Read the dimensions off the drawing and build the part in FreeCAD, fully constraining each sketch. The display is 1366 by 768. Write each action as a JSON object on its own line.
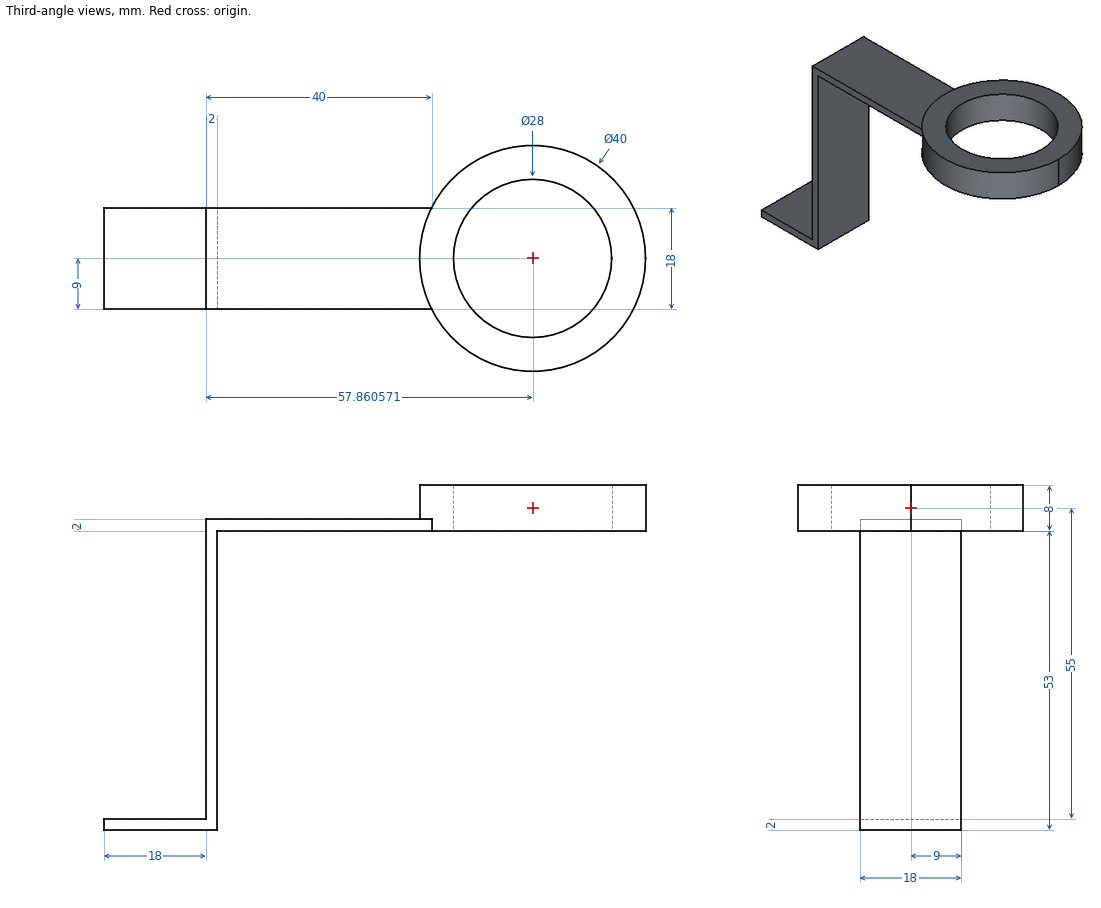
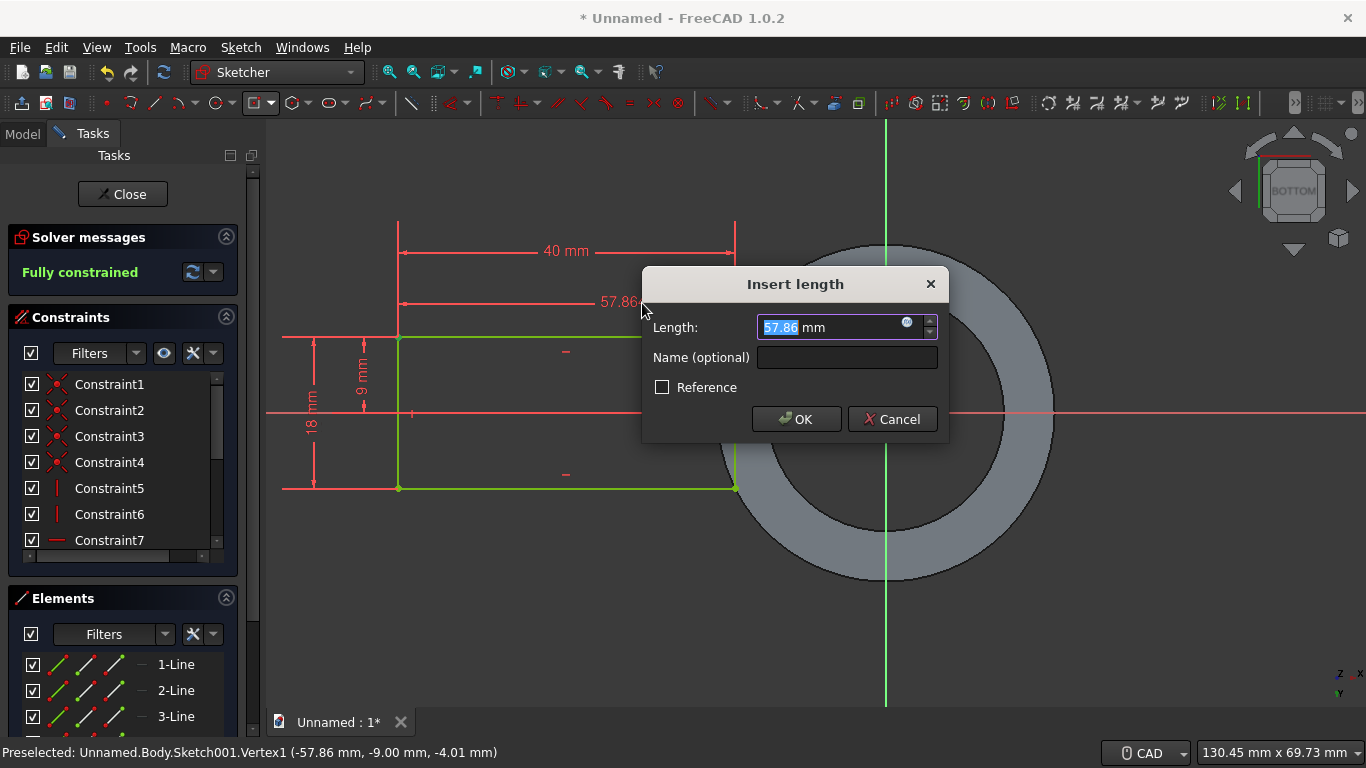
{"action": "type", "text": "57.860571"}
{"action": "key", "text": "Return"}
{"action": "key", "text": "Escape"}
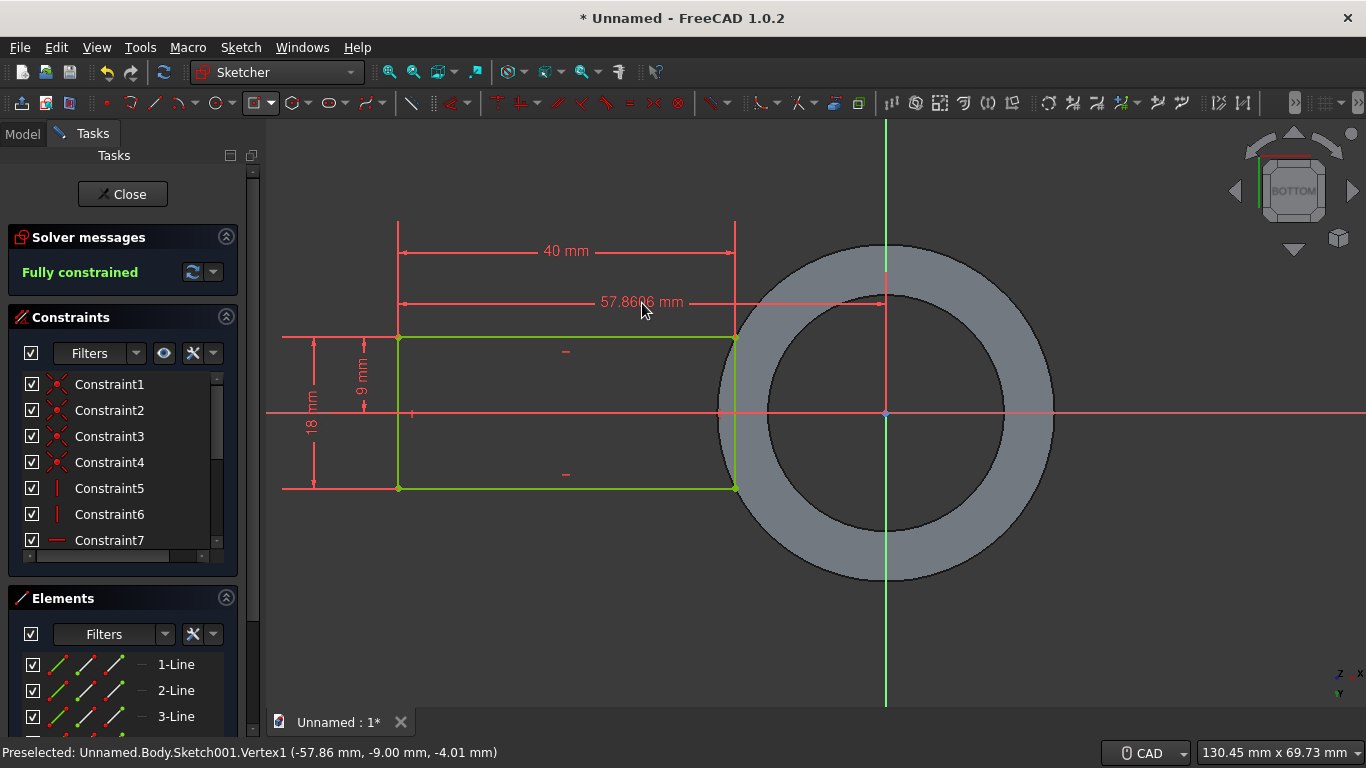
{"action": "left_click", "coordinate": [123, 194]}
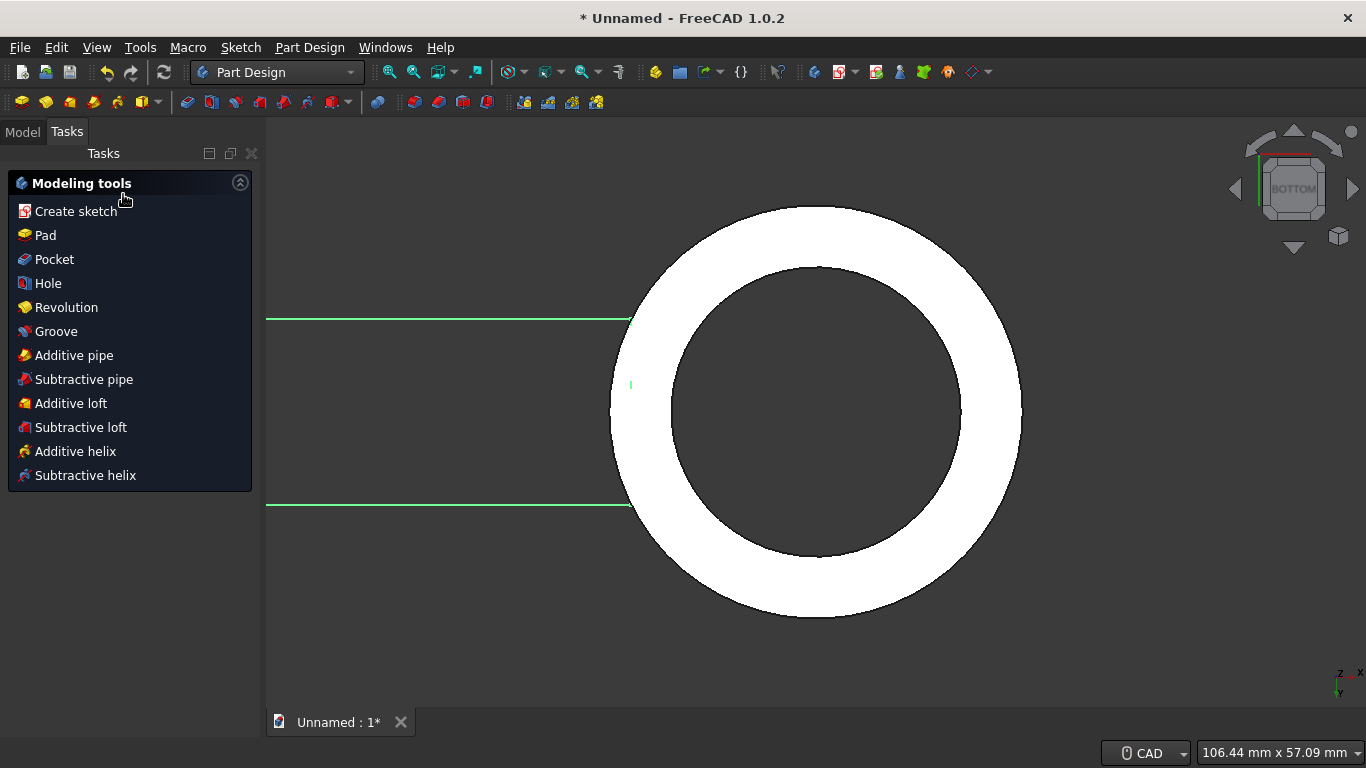
{"action": "left_click", "coordinate": [22, 102]}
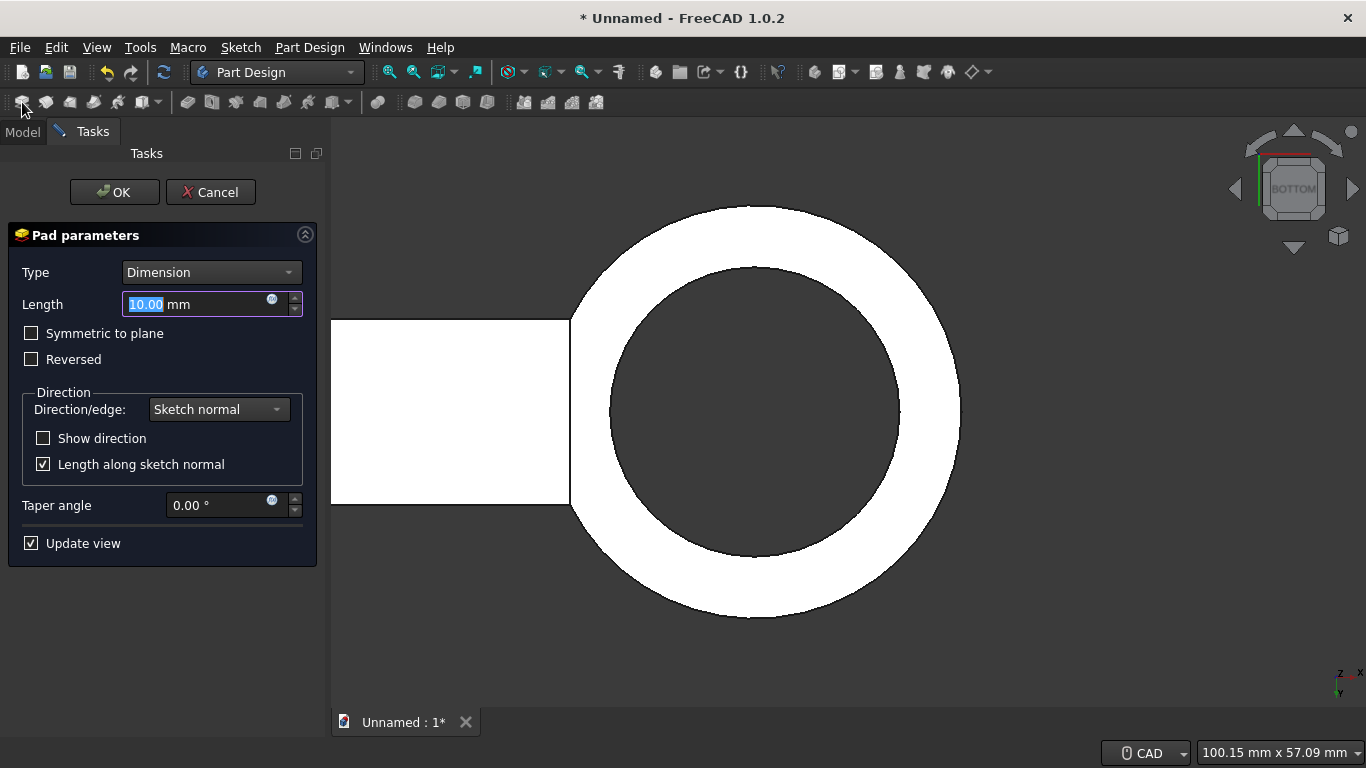
{"action": "type", "text": "2"}
{"action": "key", "text": "Tab"}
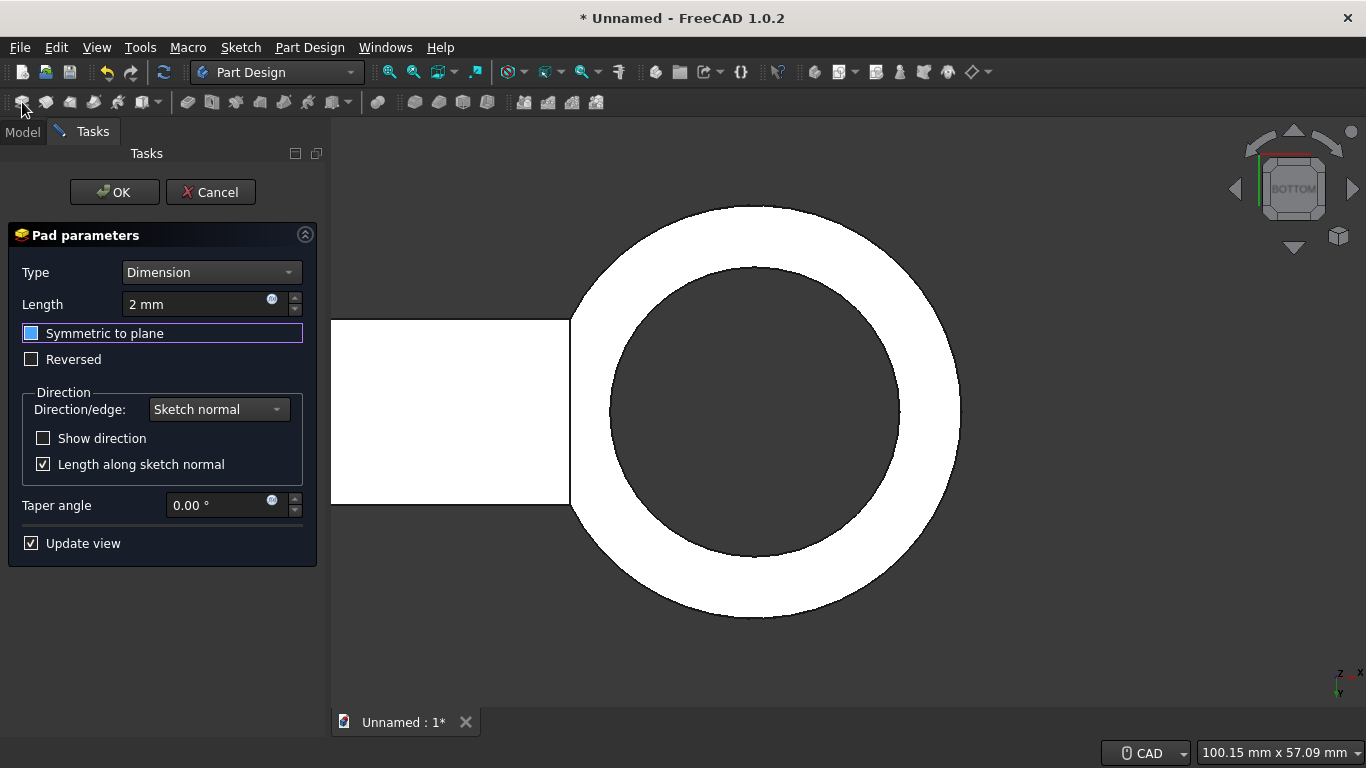
{"action": "left_click", "coordinate": [30, 359]}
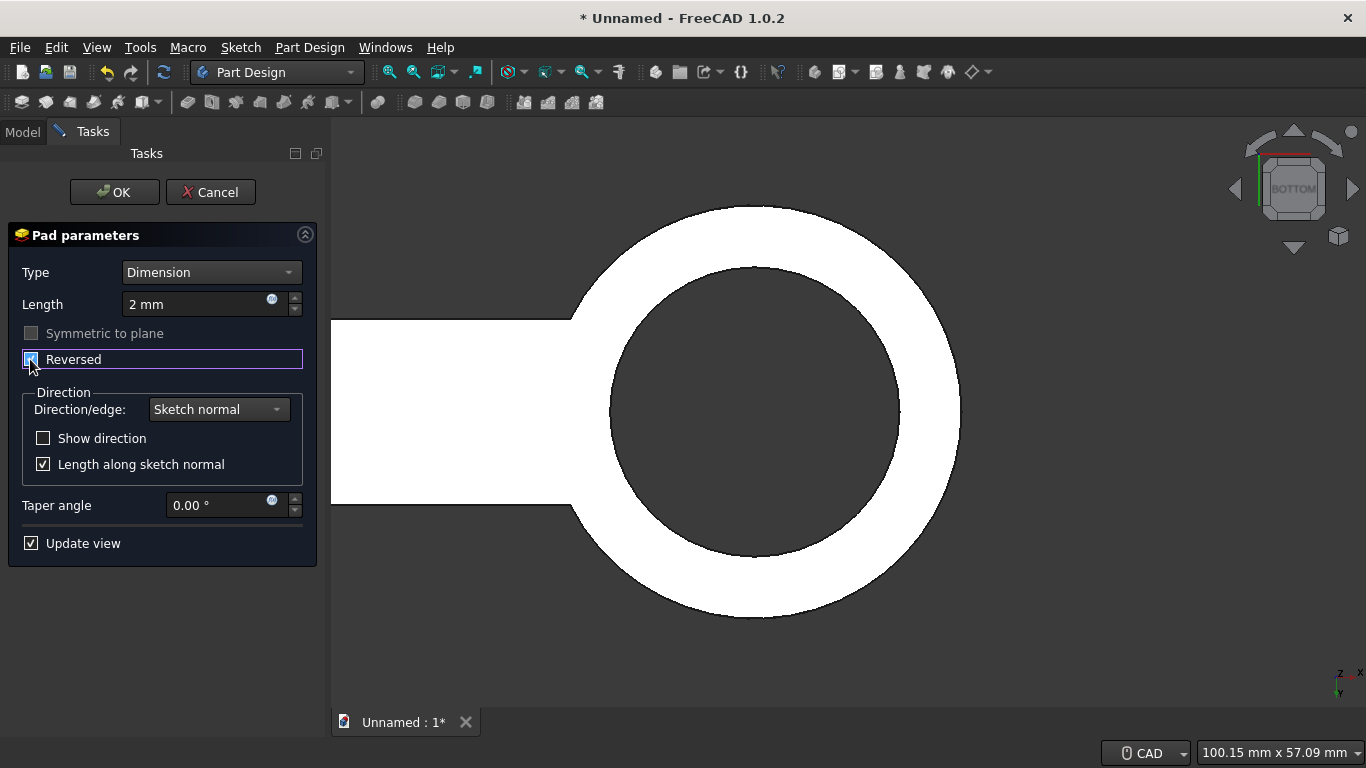
{"action": "left_click", "coordinate": [115, 192]}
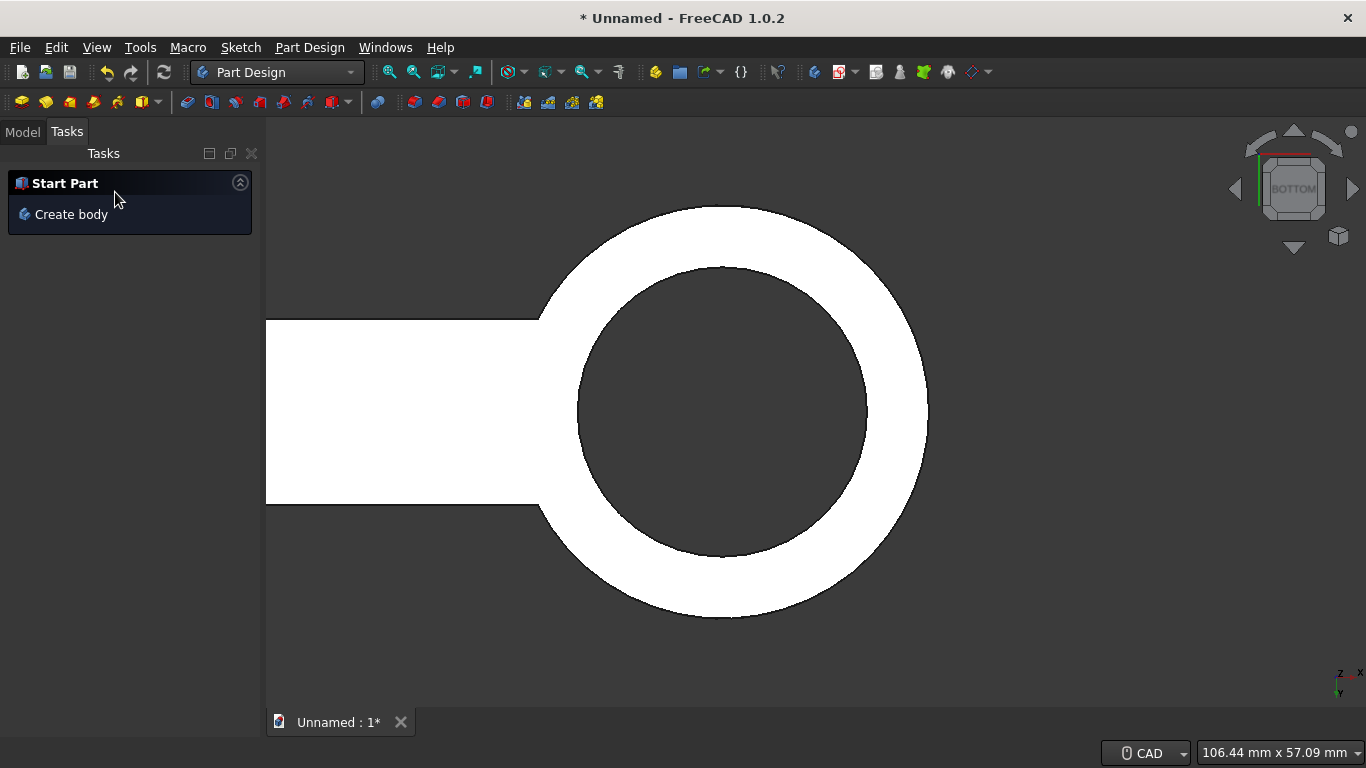
{"action": "left_click", "coordinate": [390, 72]}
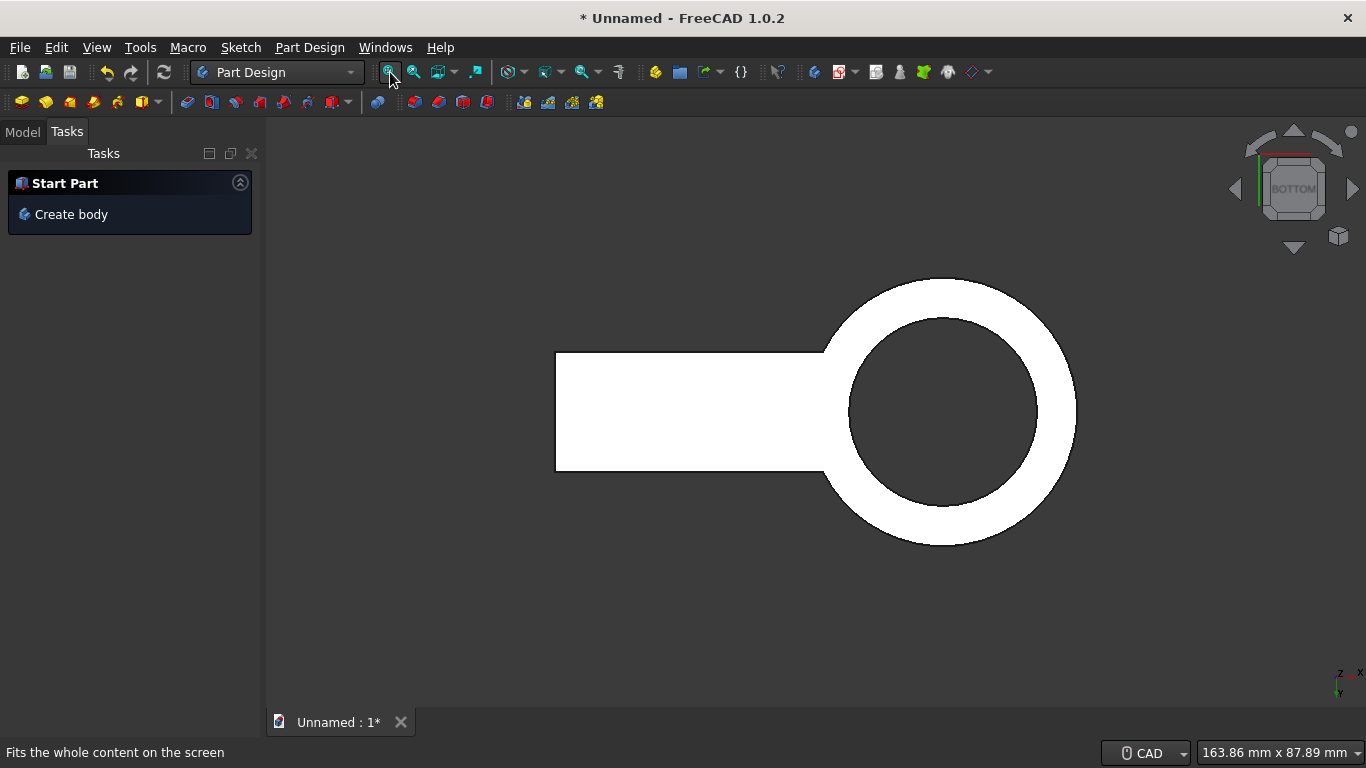
{"action": "left_click", "coordinate": [741, 411]}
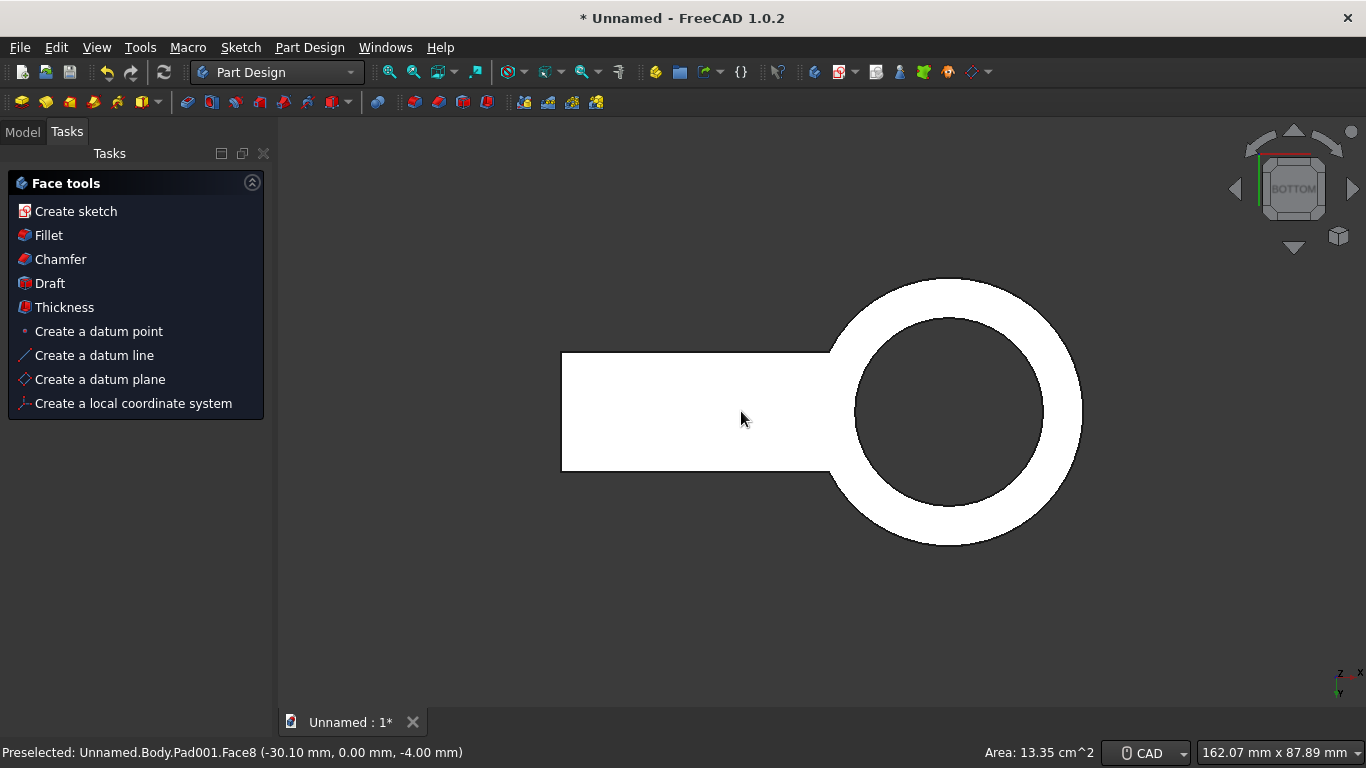
{"action": "left_click", "coordinate": [840, 72]}